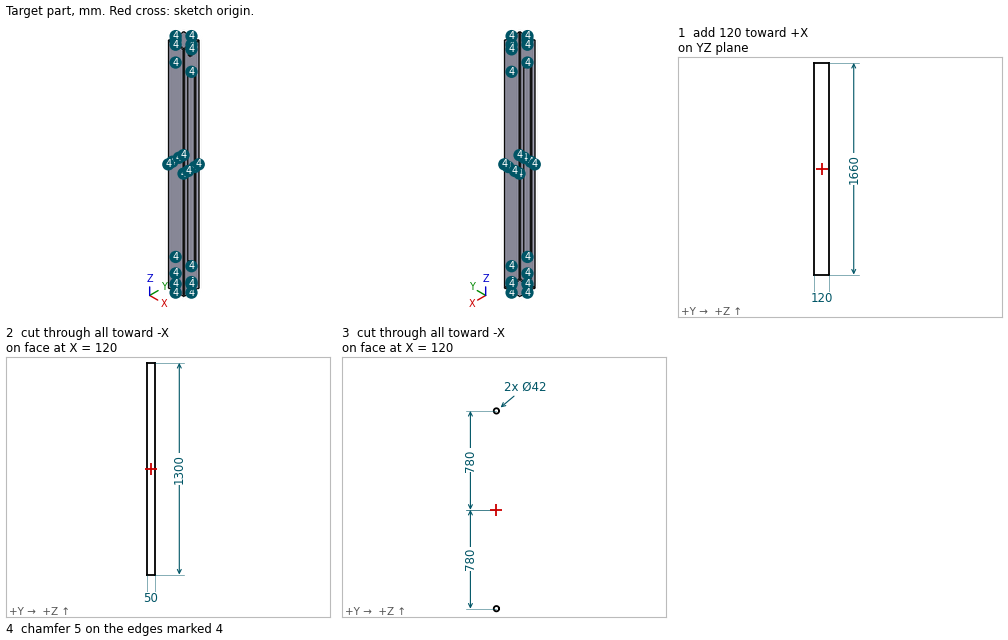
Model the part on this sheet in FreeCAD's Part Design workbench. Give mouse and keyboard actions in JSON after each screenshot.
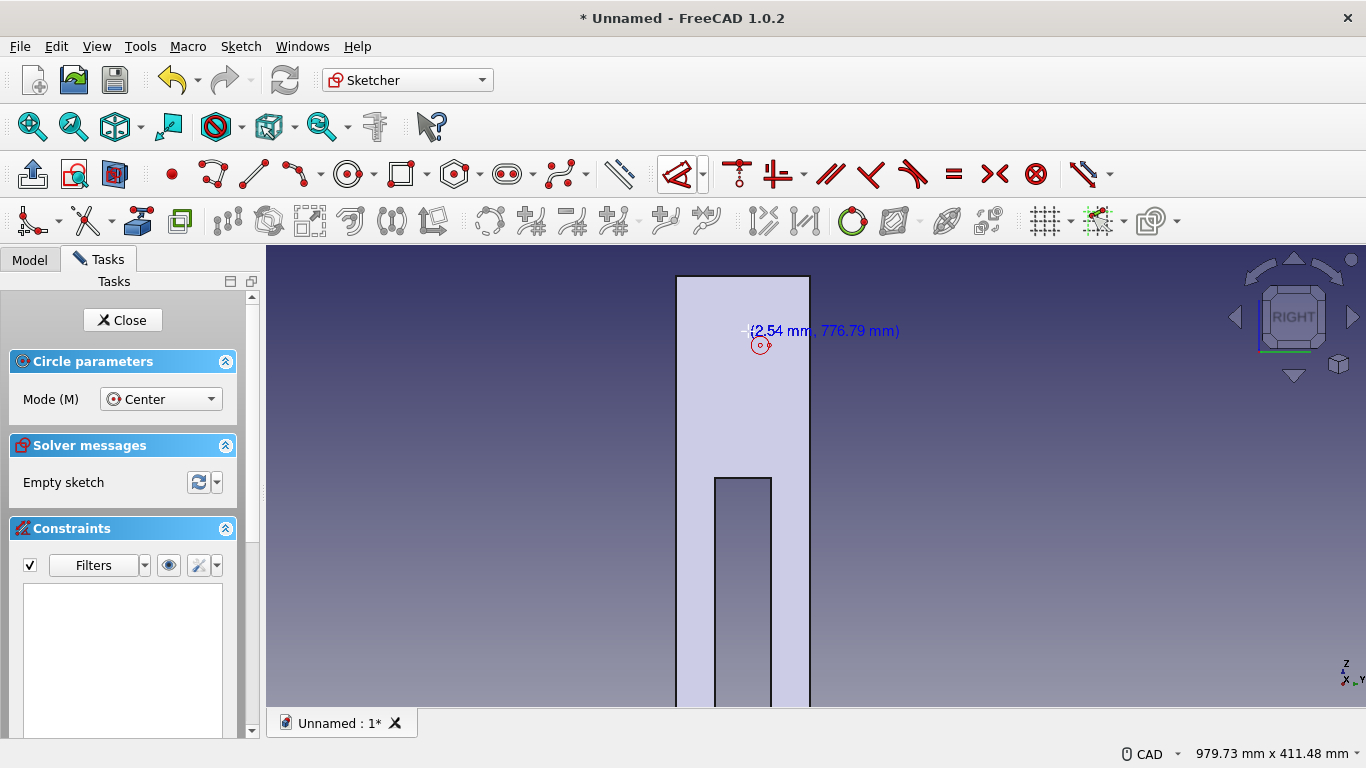
{"action": "scroll", "coordinate": [748, 331], "scroll_direction": "down", "scroll_amount": 9}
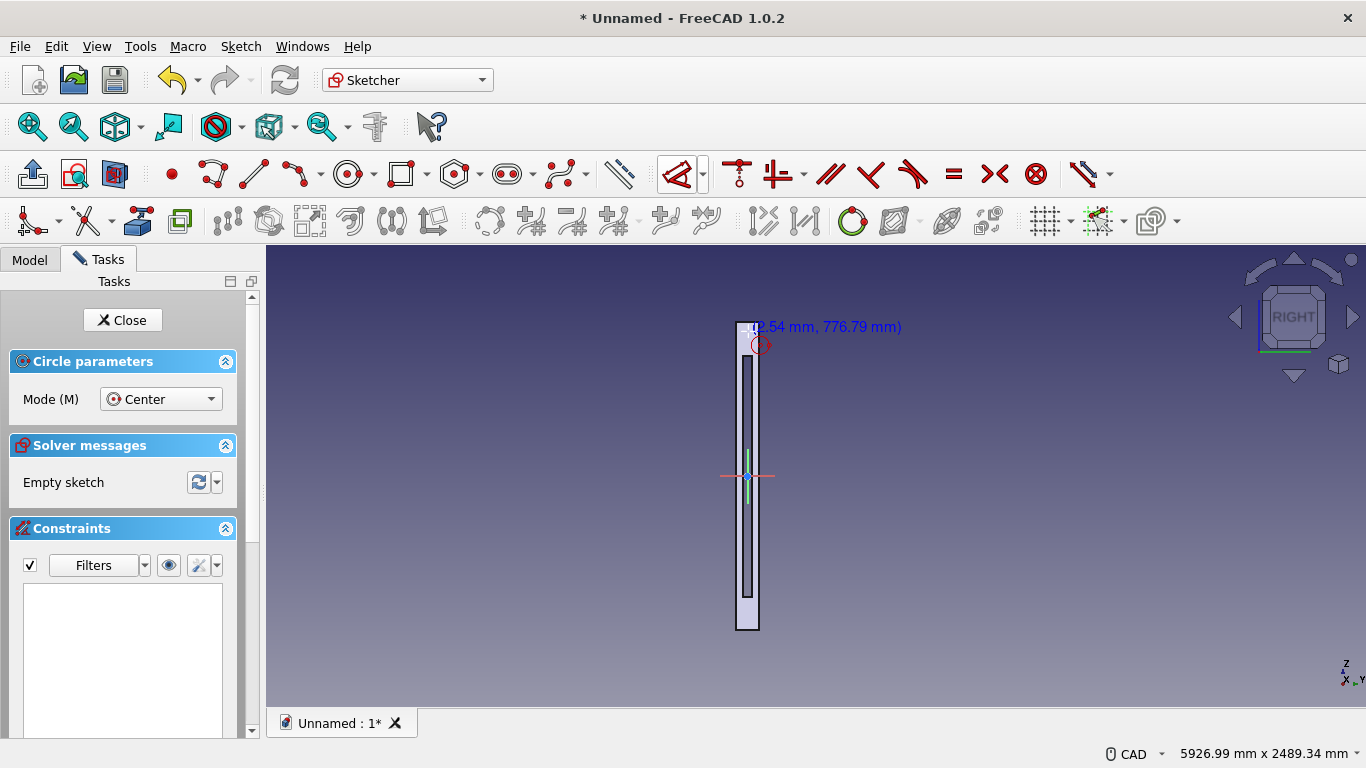
{"action": "left_click", "coordinate": [748, 331]}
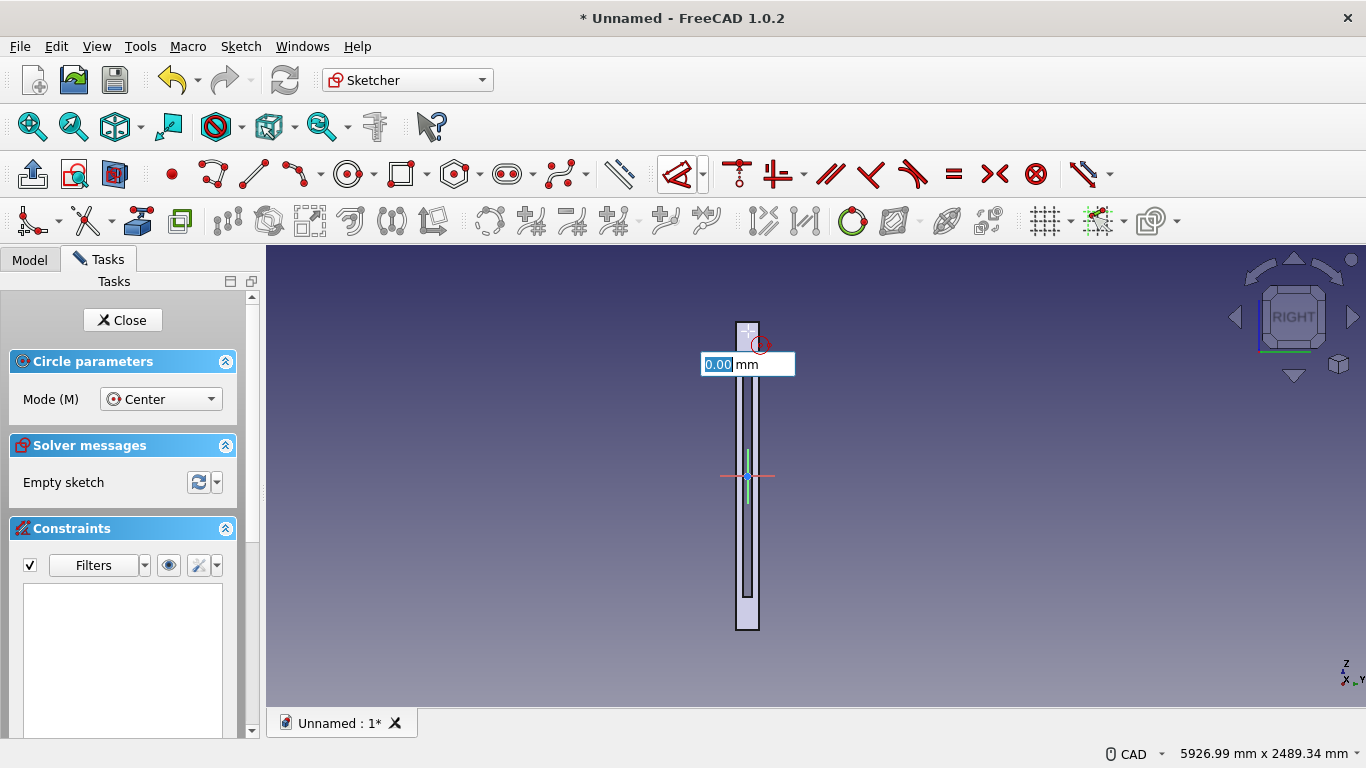
{"action": "scroll", "coordinate": [751, 330], "scroll_direction": "up", "scroll_amount": 8}
{"action": "mouse_move", "coordinate": [750, 330]}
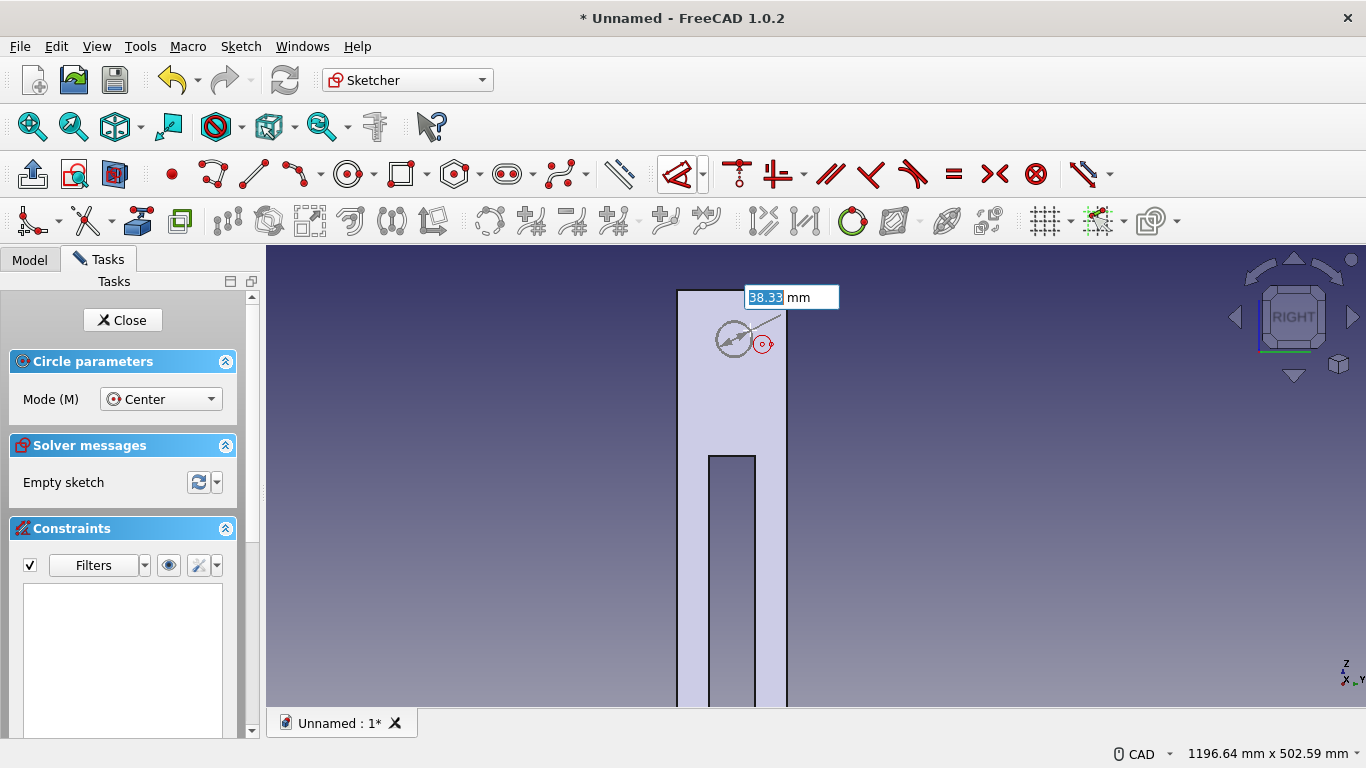
{"action": "type", "text": "42"}
{"action": "key", "text": "Return"}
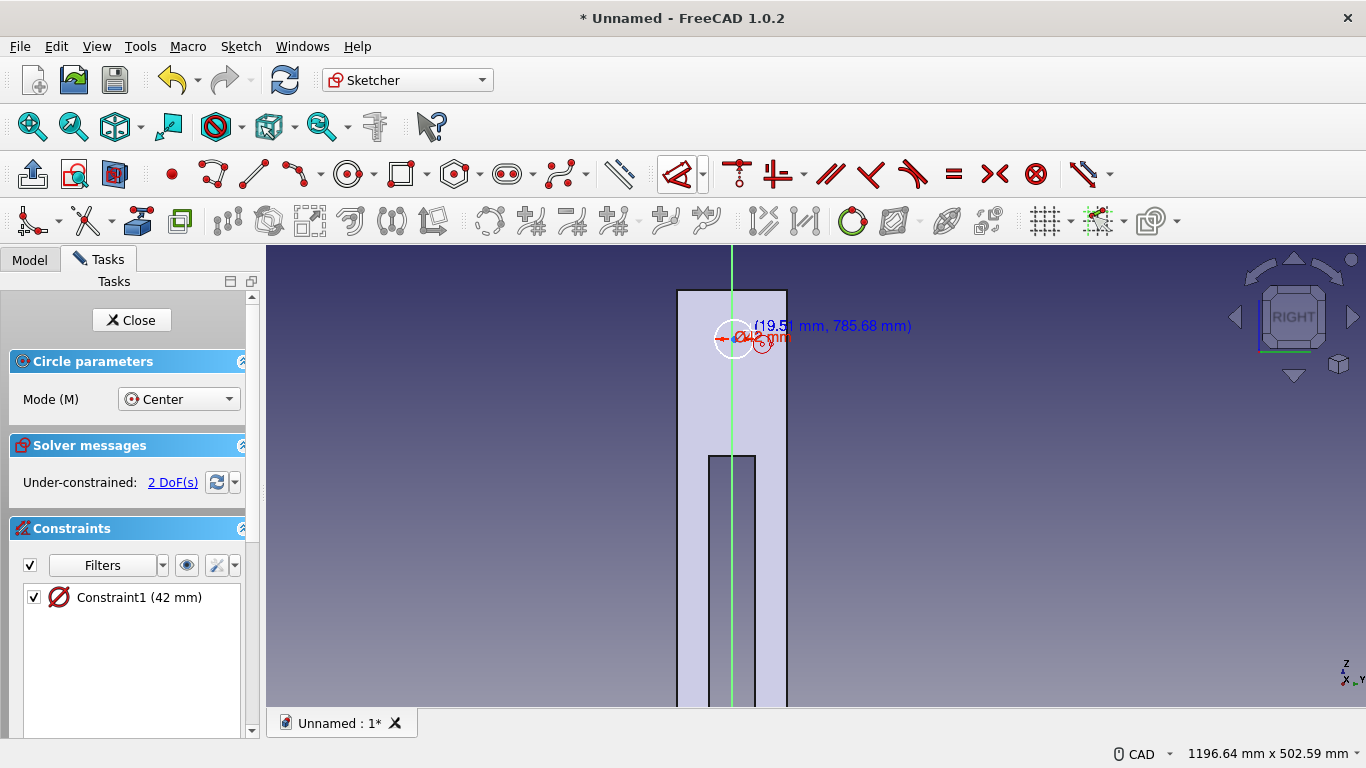
{"action": "scroll", "coordinate": [751, 330], "scroll_direction": "down", "scroll_amount": 8}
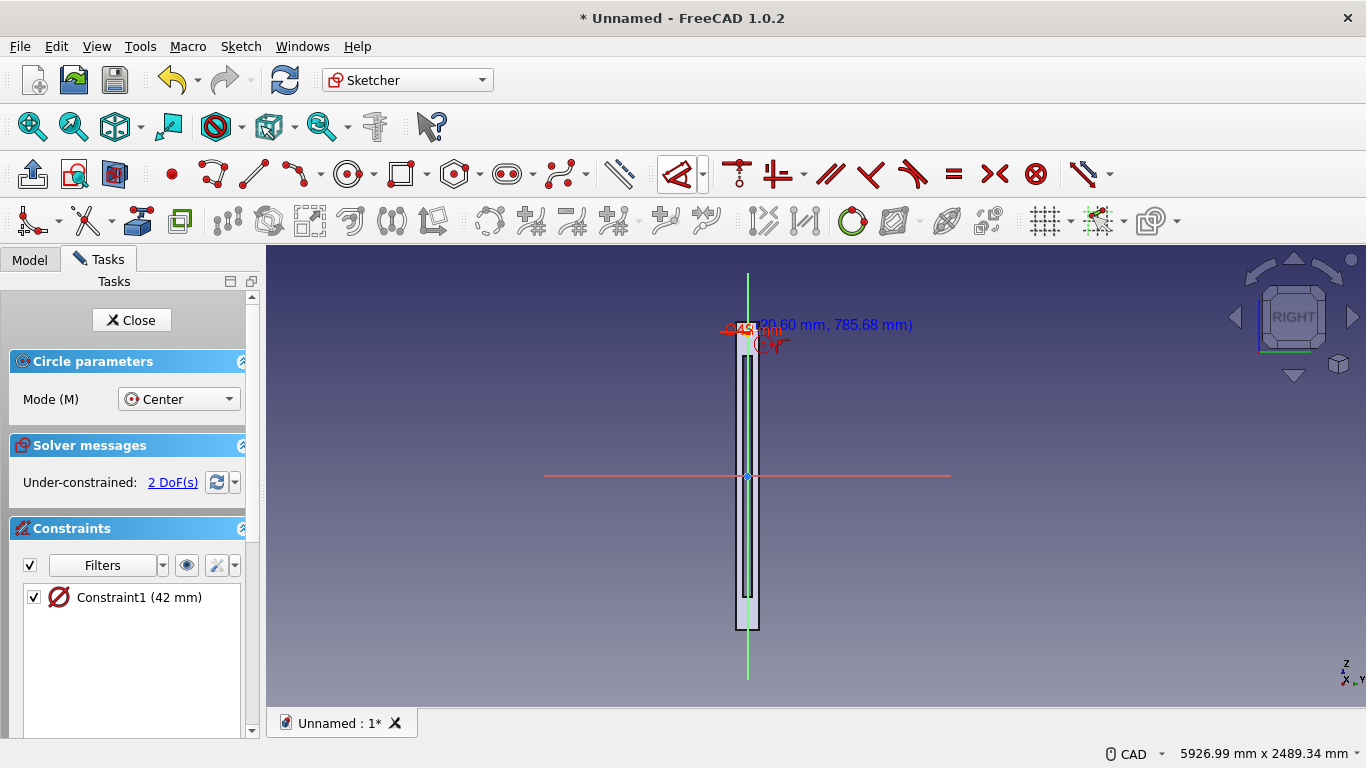
{"action": "scroll", "coordinate": [748, 621], "scroll_direction": "up", "scroll_amount": 9}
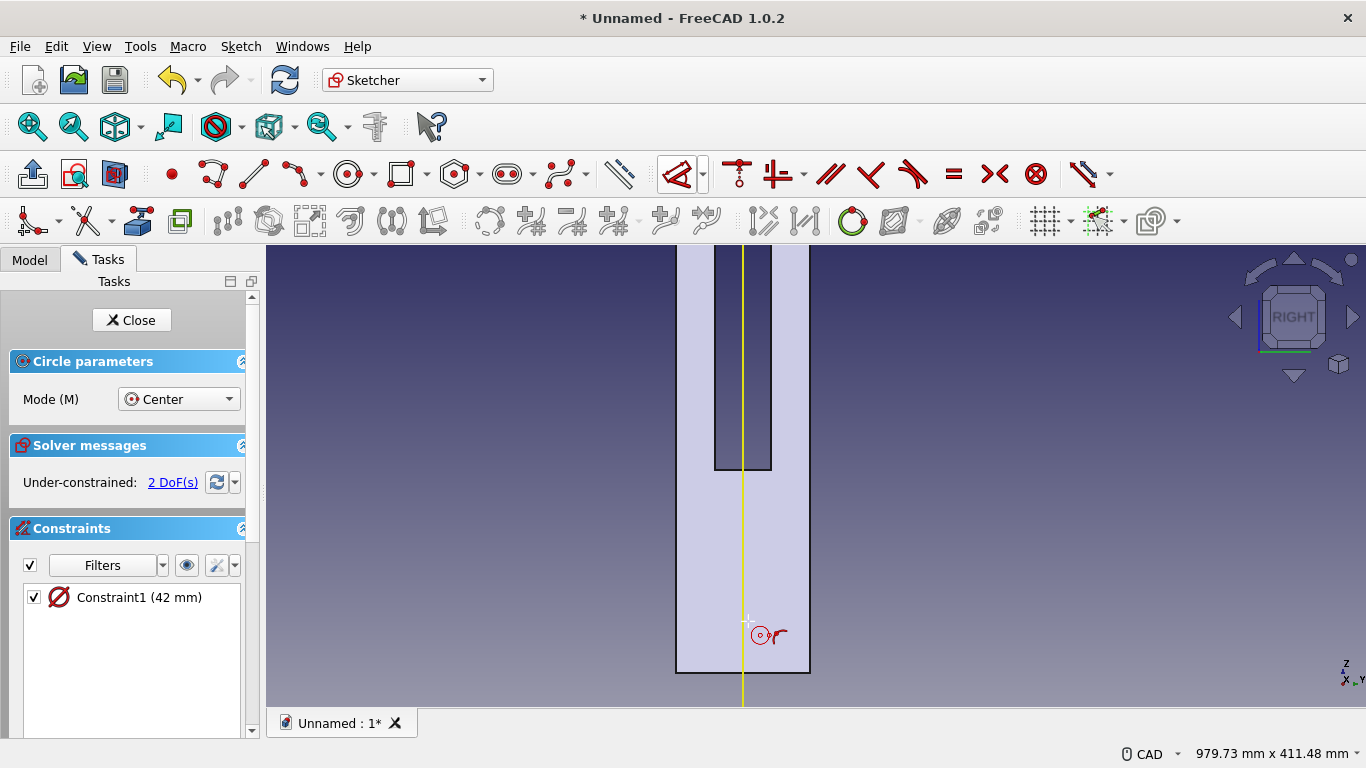
{"action": "scroll", "coordinate": [748, 622], "scroll_direction": "down", "scroll_amount": 9}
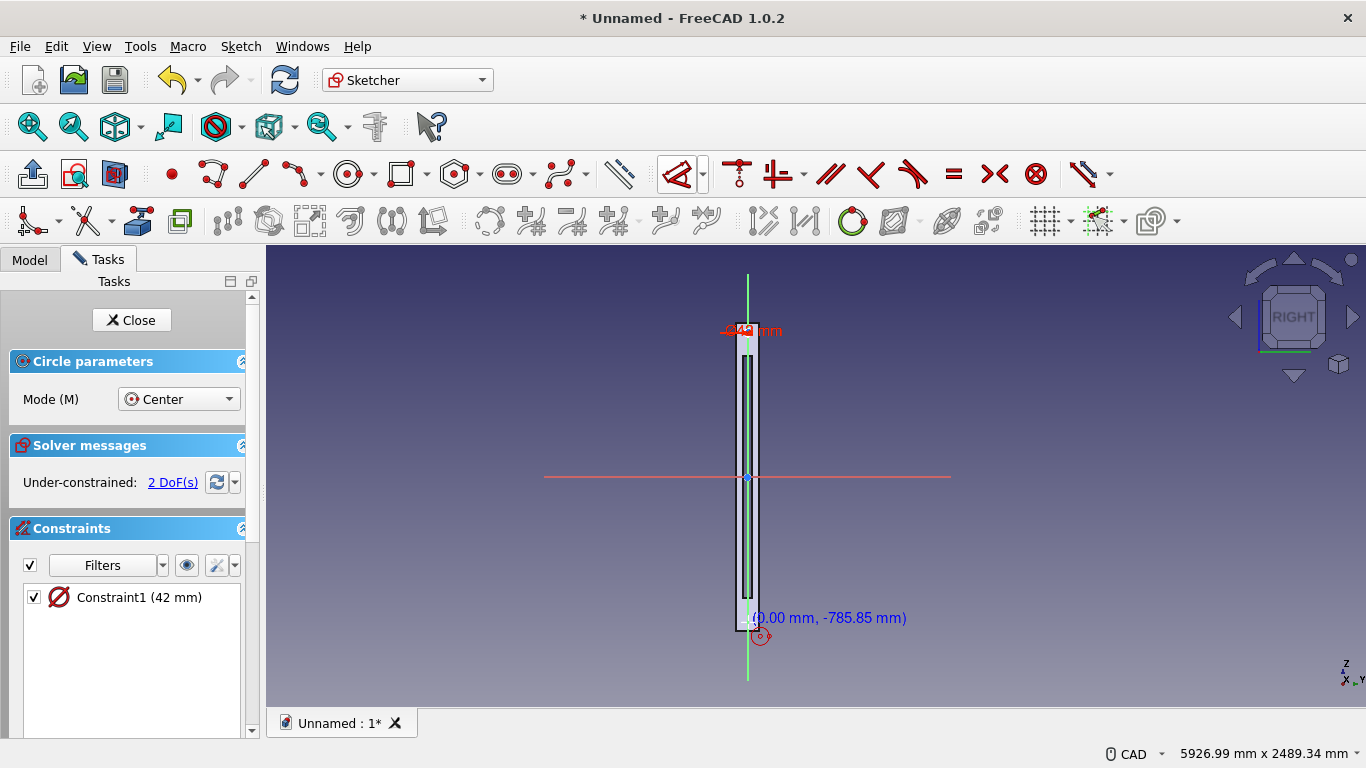
{"action": "left_click", "coordinate": [748, 622]}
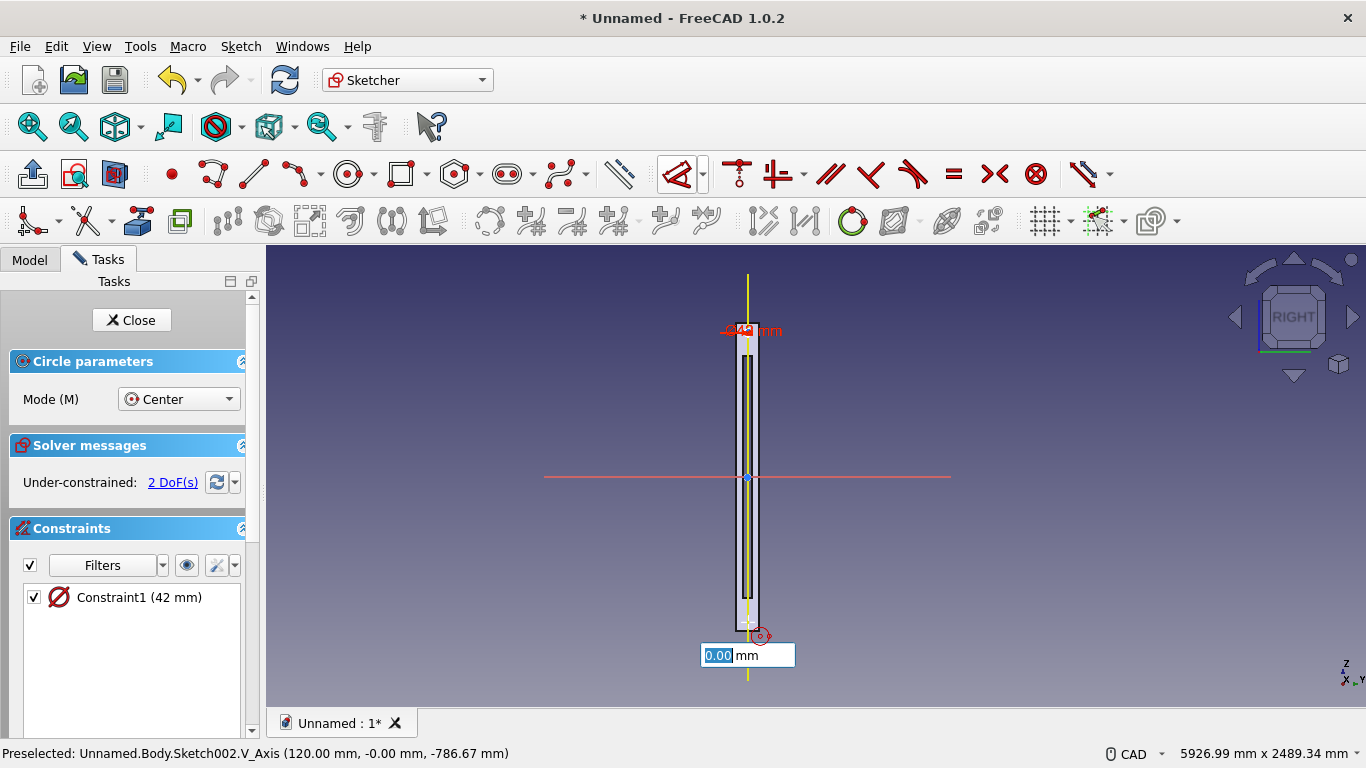
{"action": "scroll", "coordinate": [751, 620], "scroll_direction": "up", "scroll_amount": 8}
{"action": "mouse_move", "coordinate": [750, 619]}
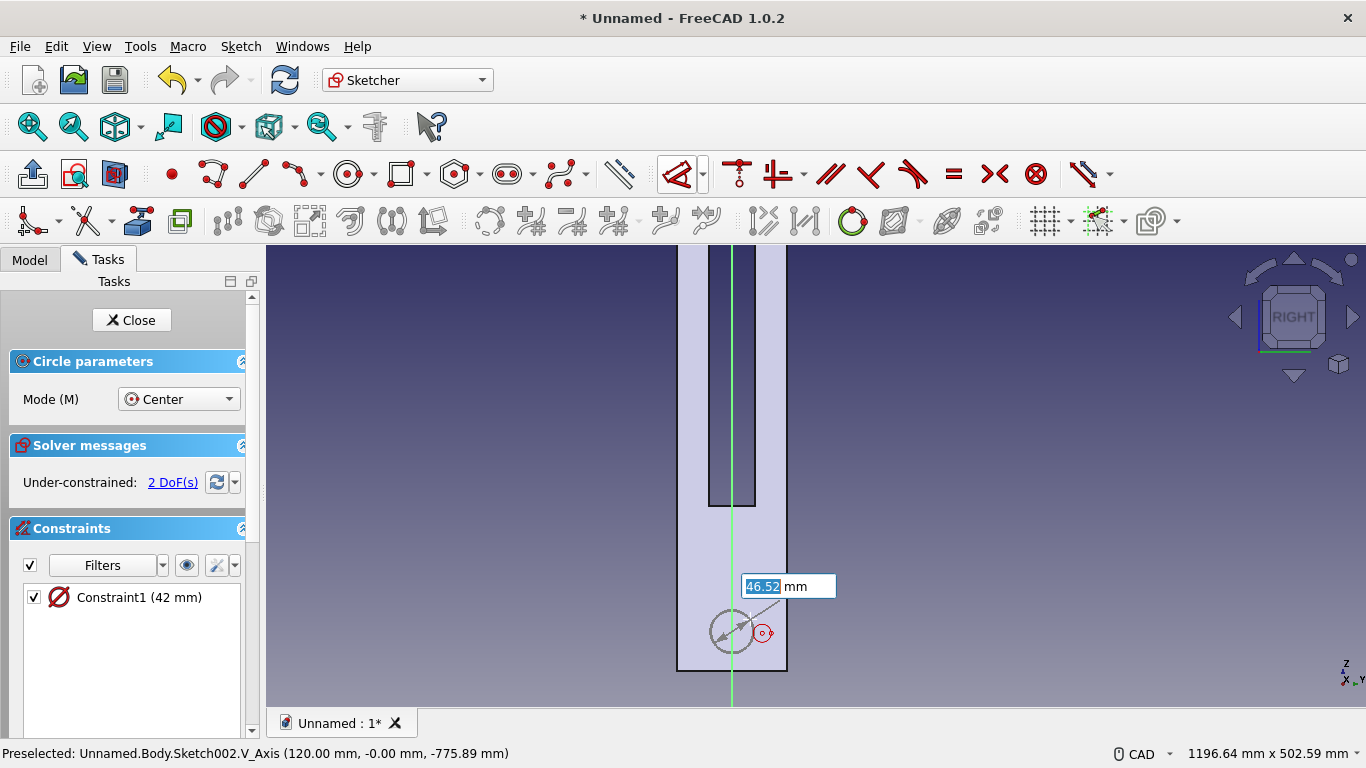
{"action": "type", "text": "42"}
{"action": "key", "text": "Return"}
{"action": "key", "text": "Escape"}